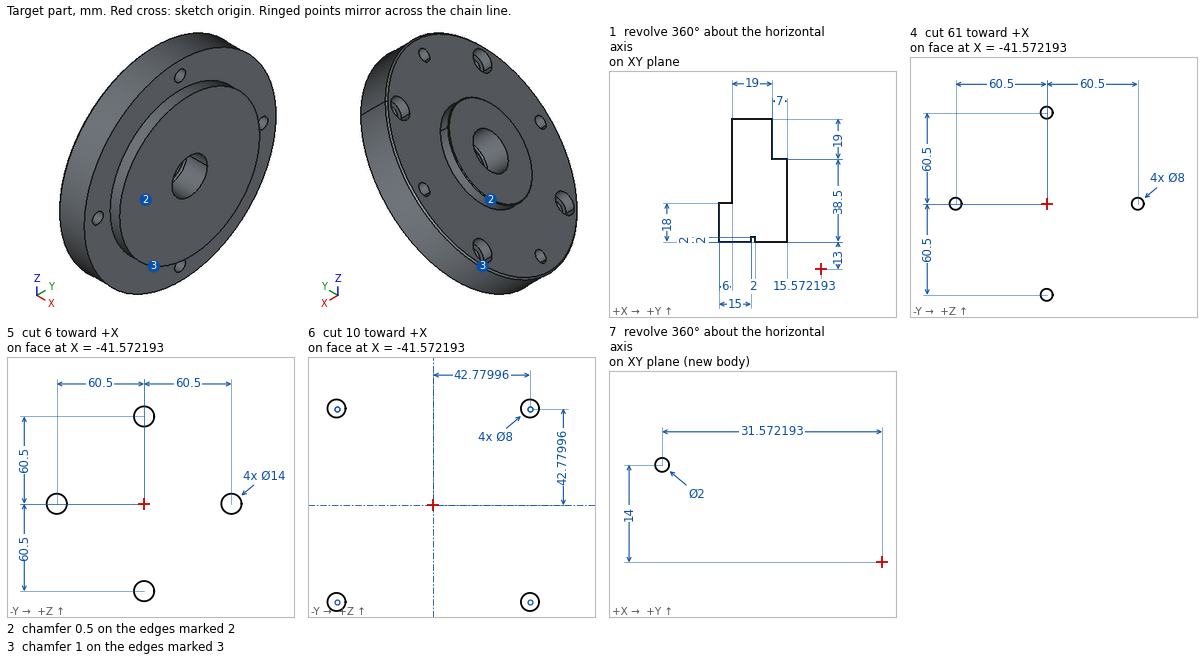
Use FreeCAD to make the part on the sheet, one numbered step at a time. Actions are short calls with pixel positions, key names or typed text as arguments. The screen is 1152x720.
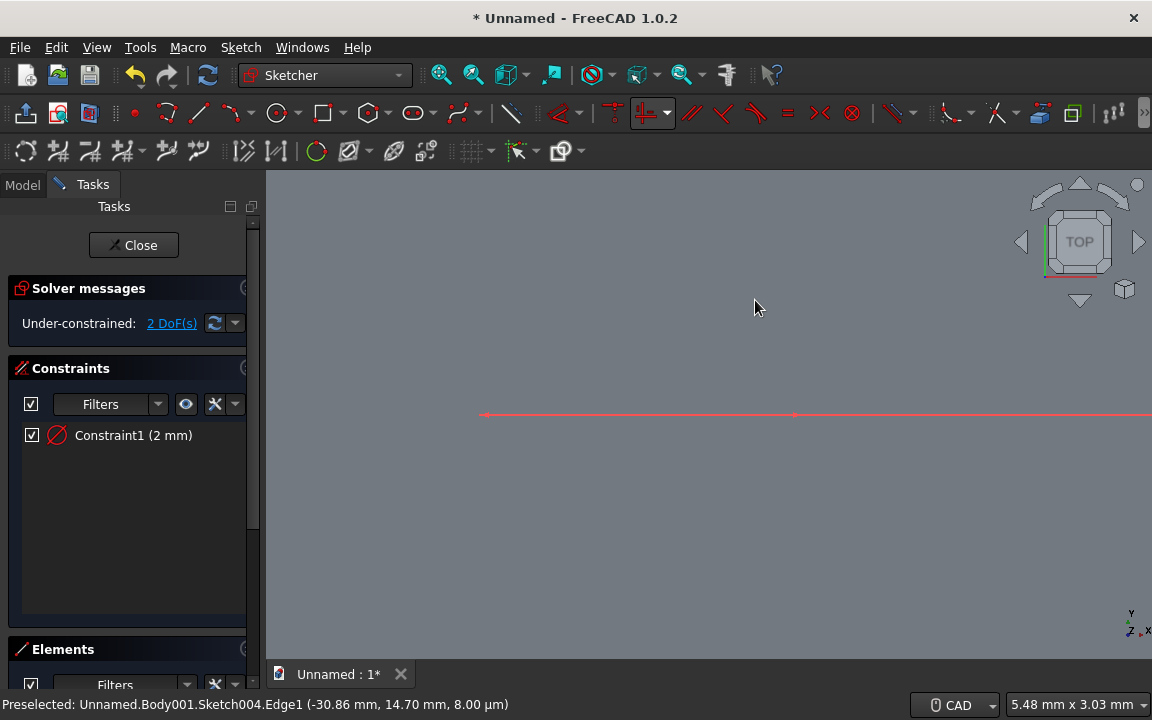
click(558, 114)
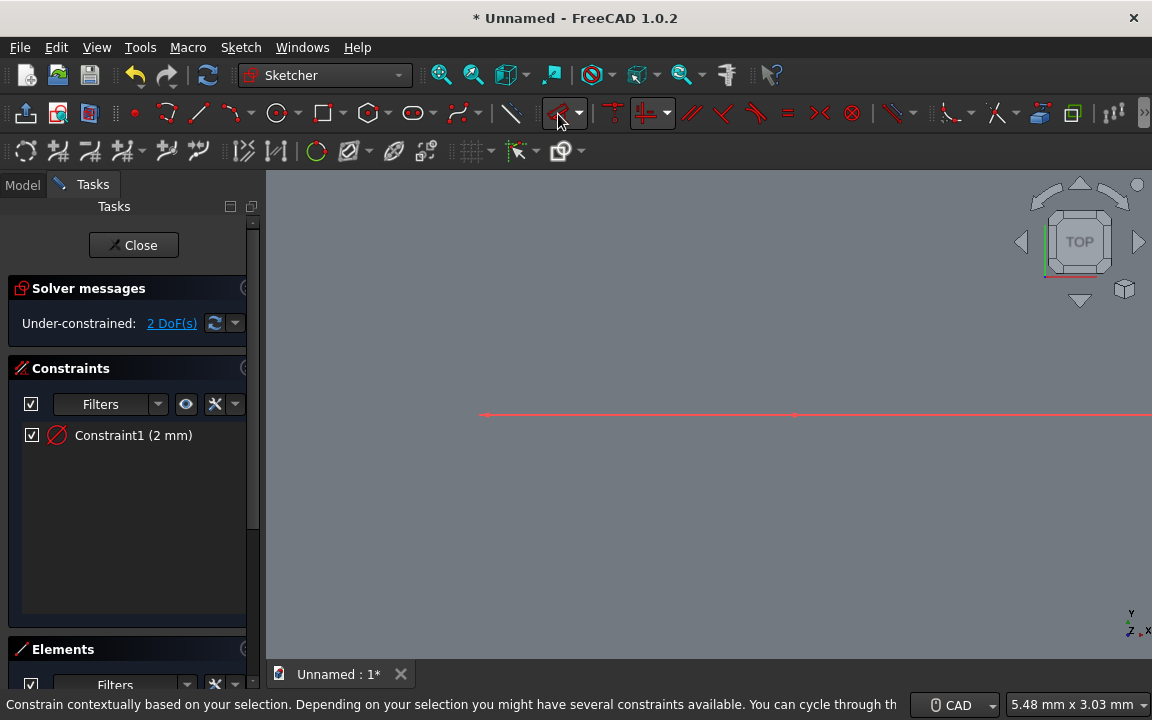
click(641, 415)
click(607, 523)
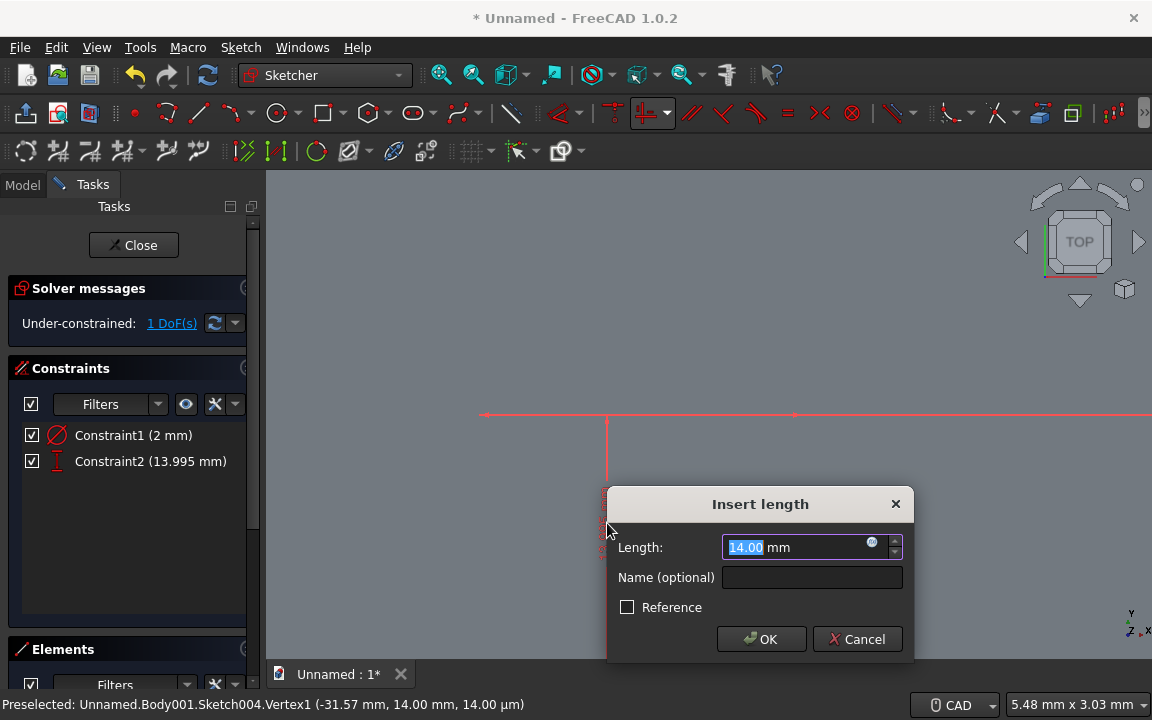
text(14)
key(Return)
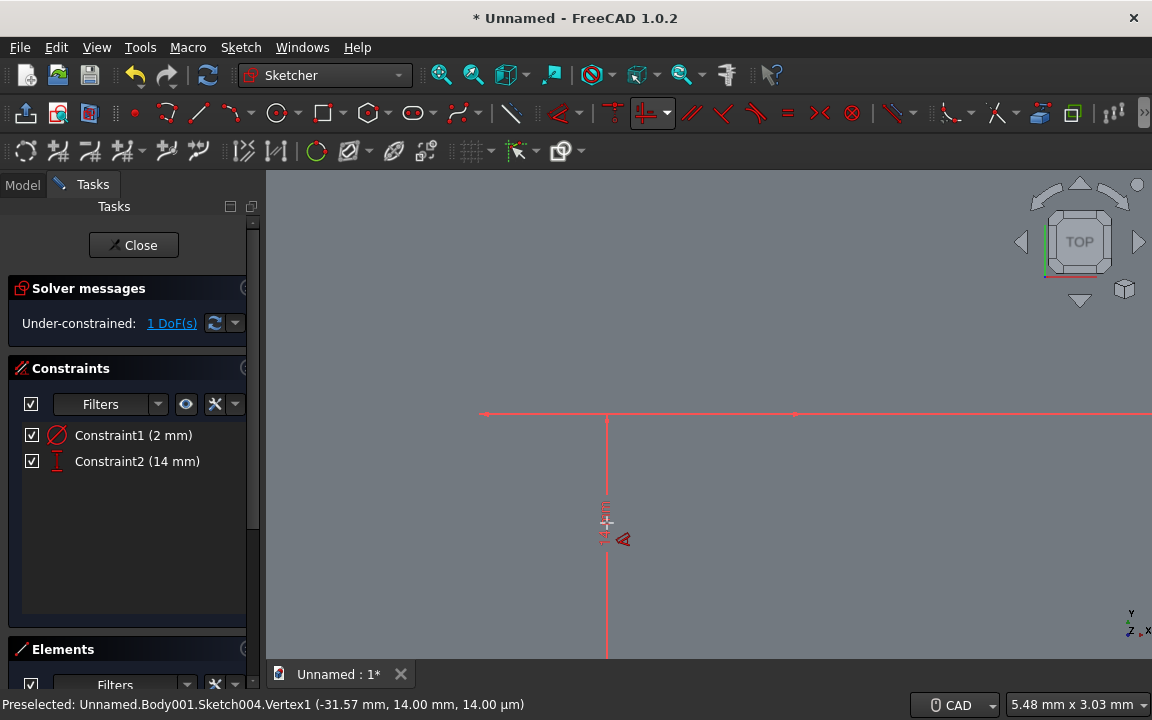
click(641, 414)
click(814, 380)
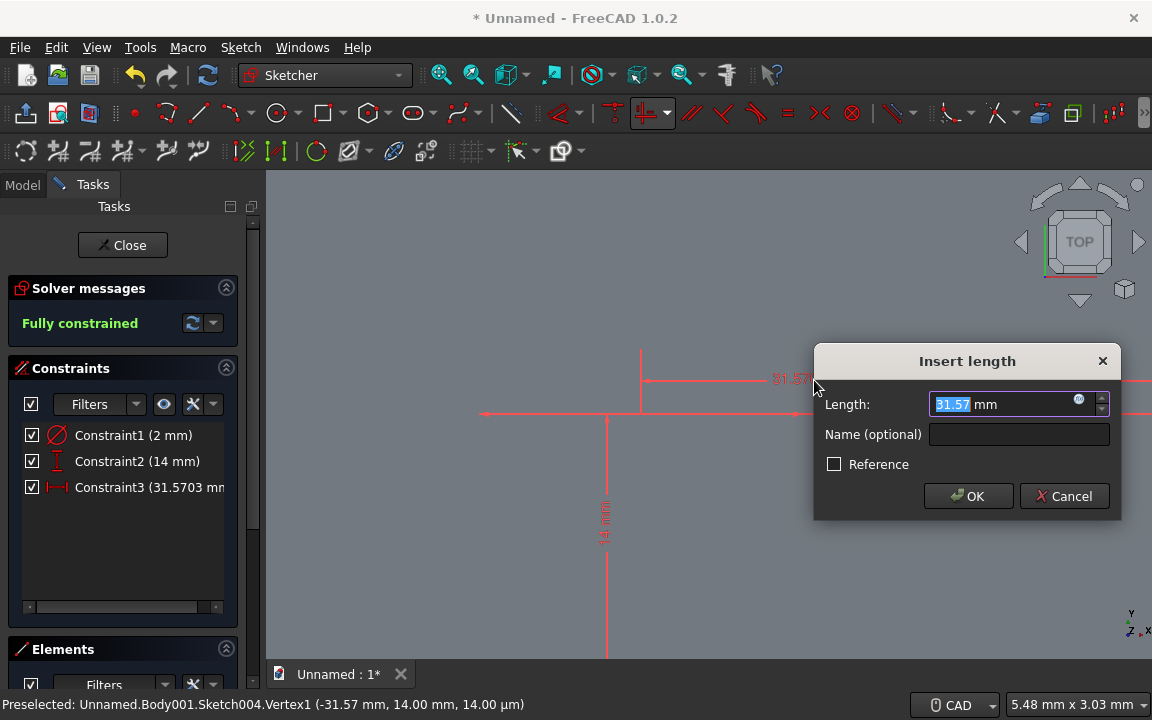
text(31.572193)
key(Return)
key(Escape)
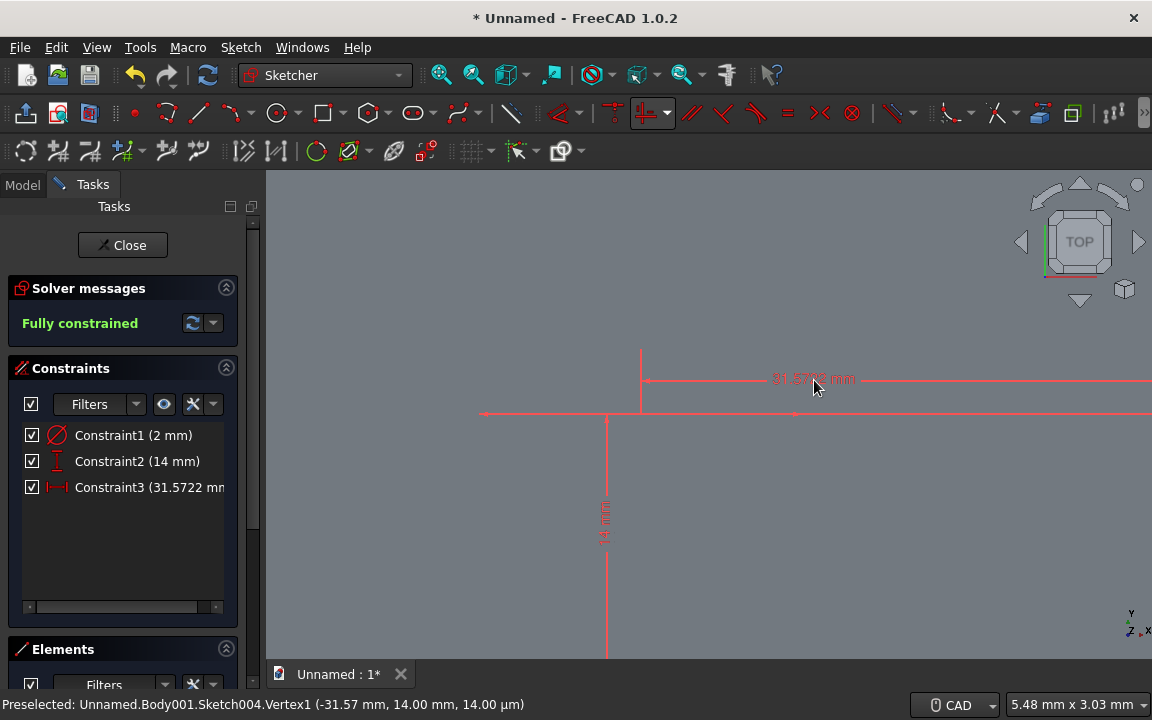
click(123, 245)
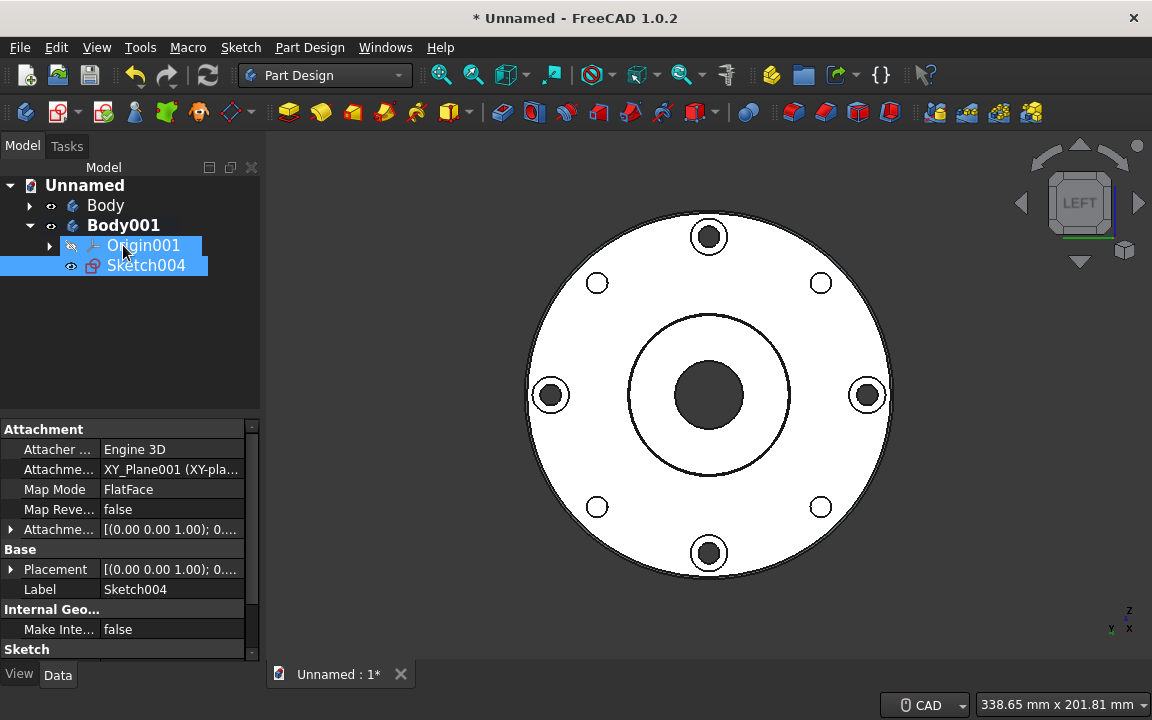
click(322, 112)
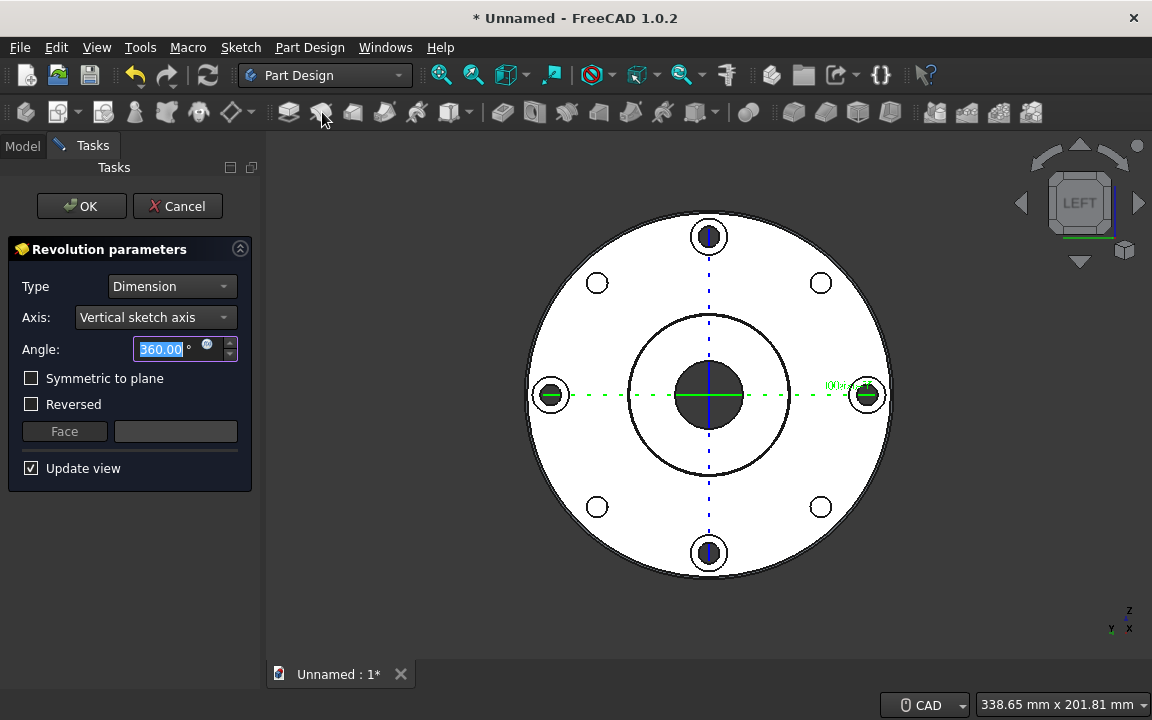
click(156, 318)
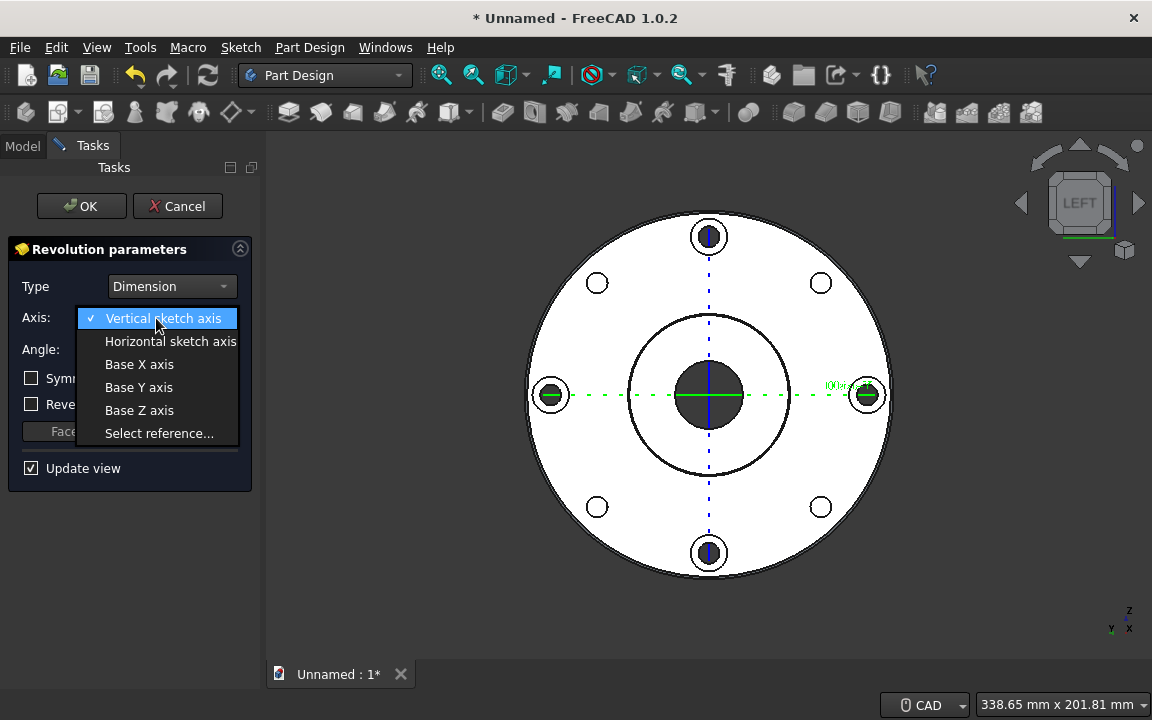
click(156, 342)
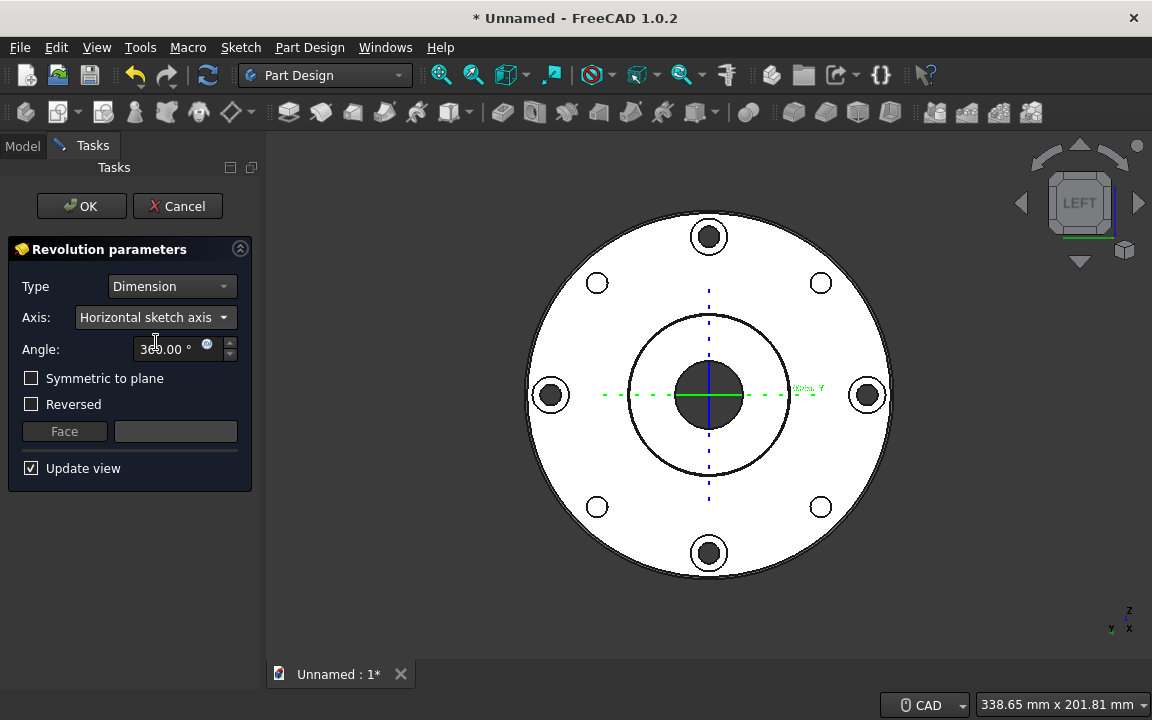
click(82, 206)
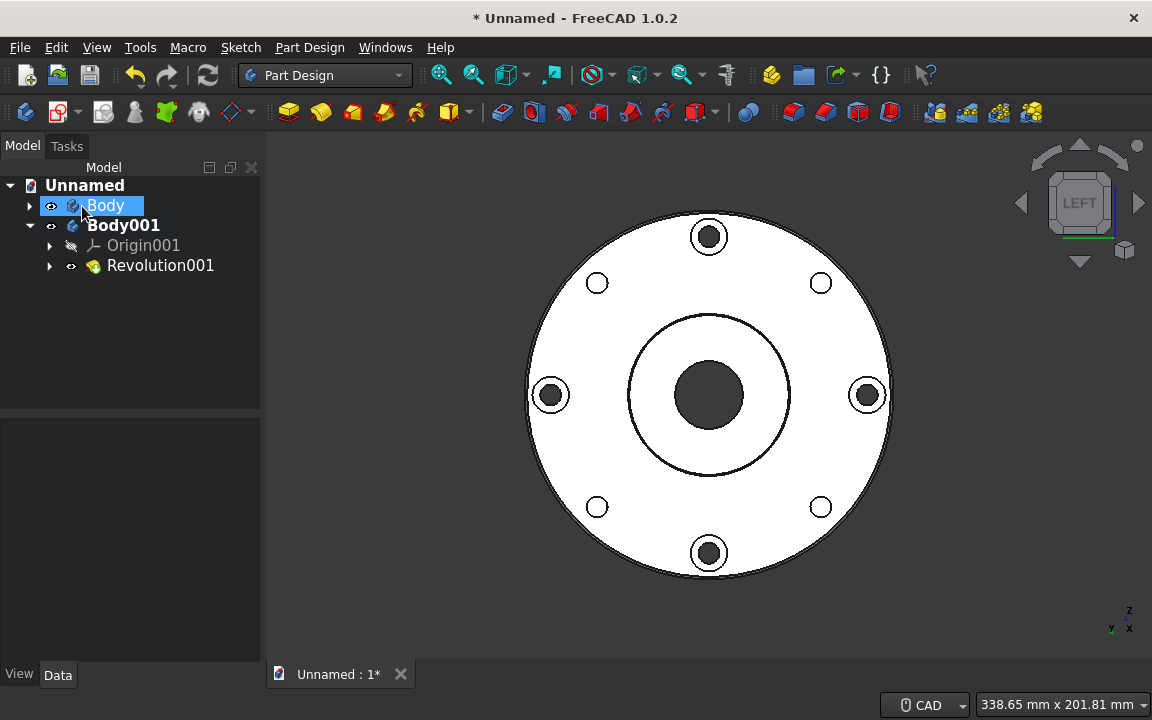
key(0)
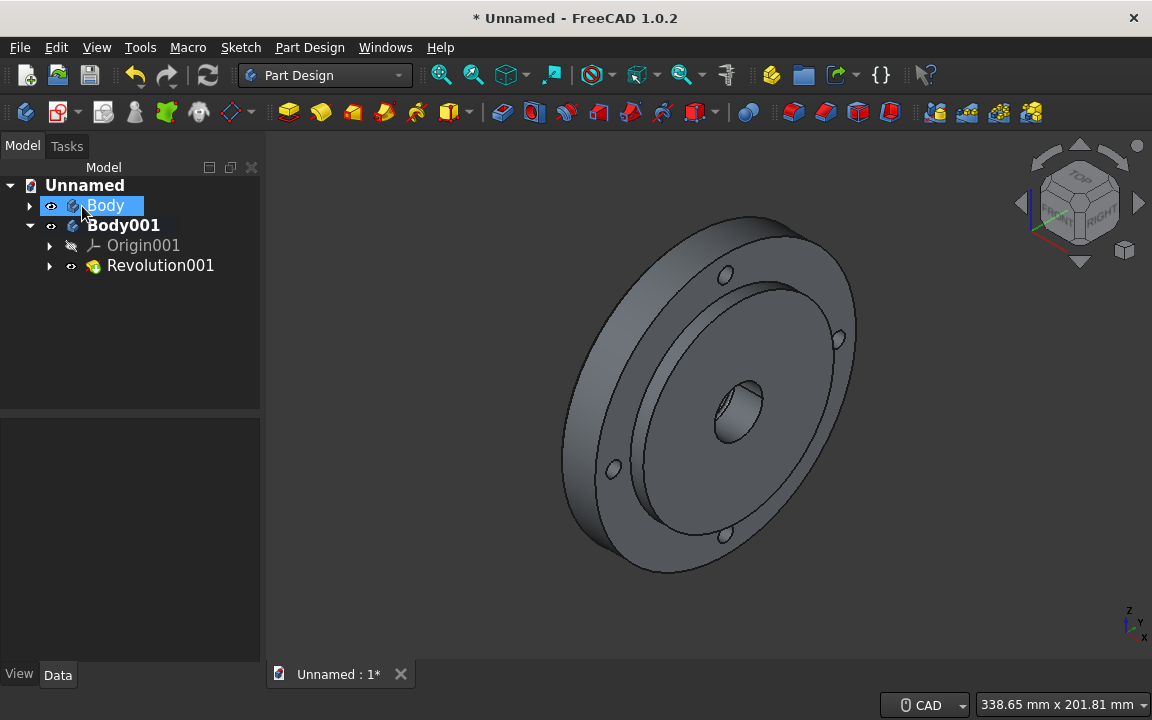
click(442, 76)